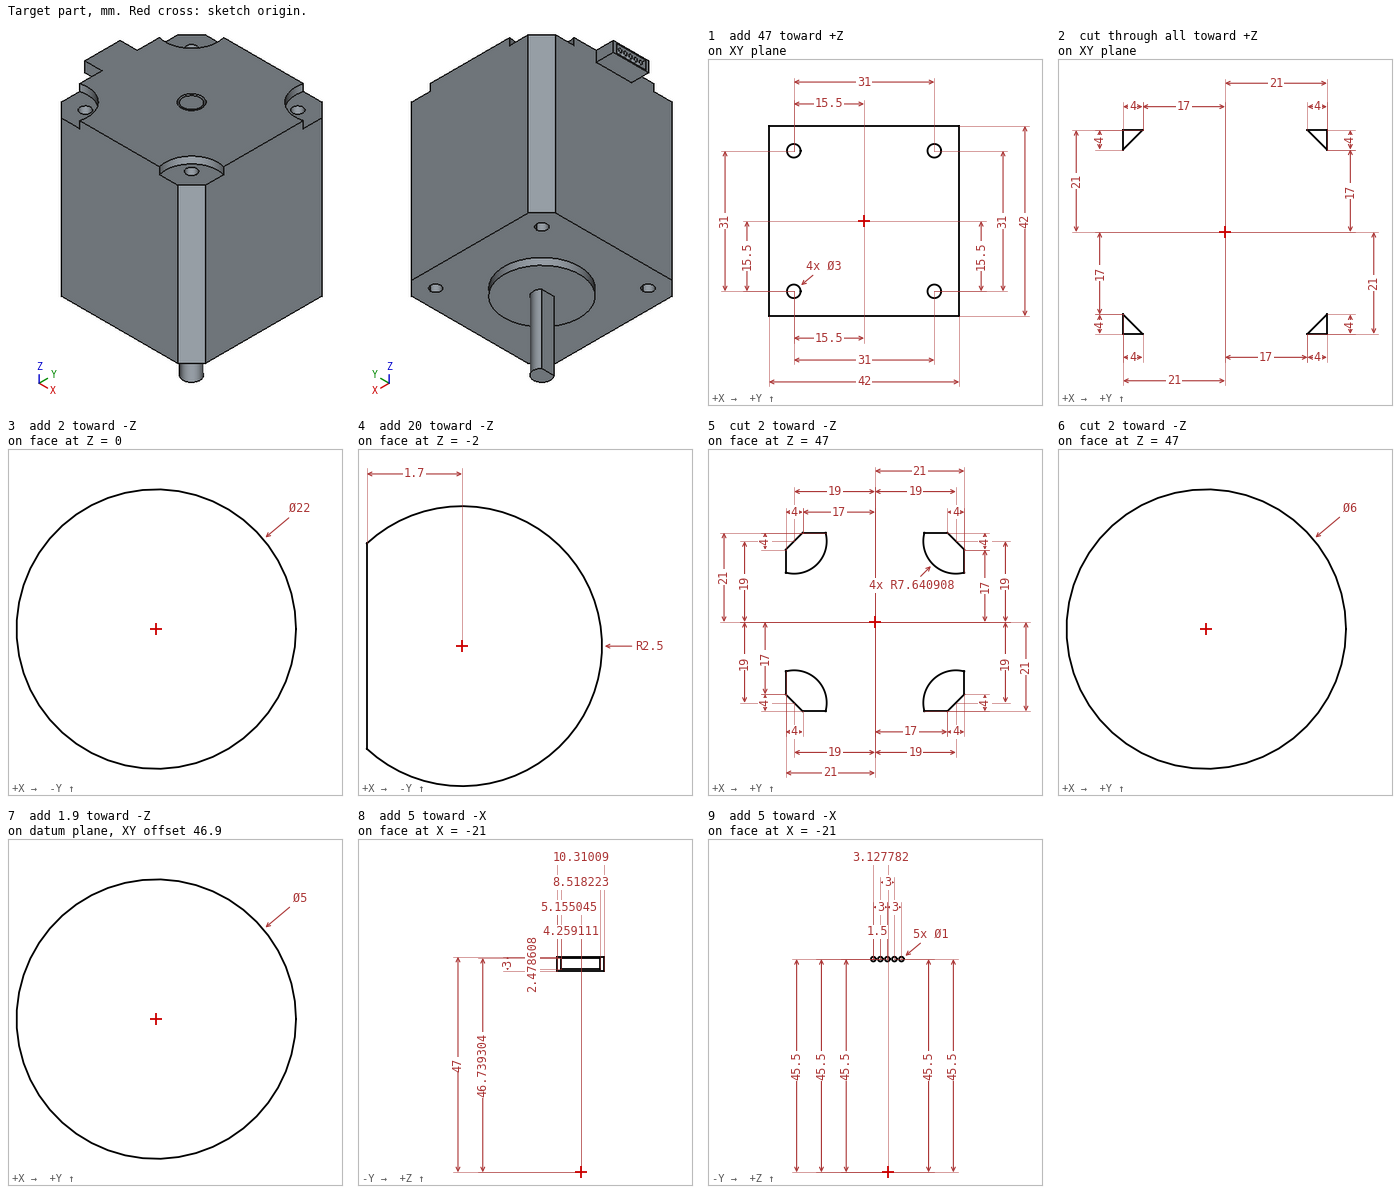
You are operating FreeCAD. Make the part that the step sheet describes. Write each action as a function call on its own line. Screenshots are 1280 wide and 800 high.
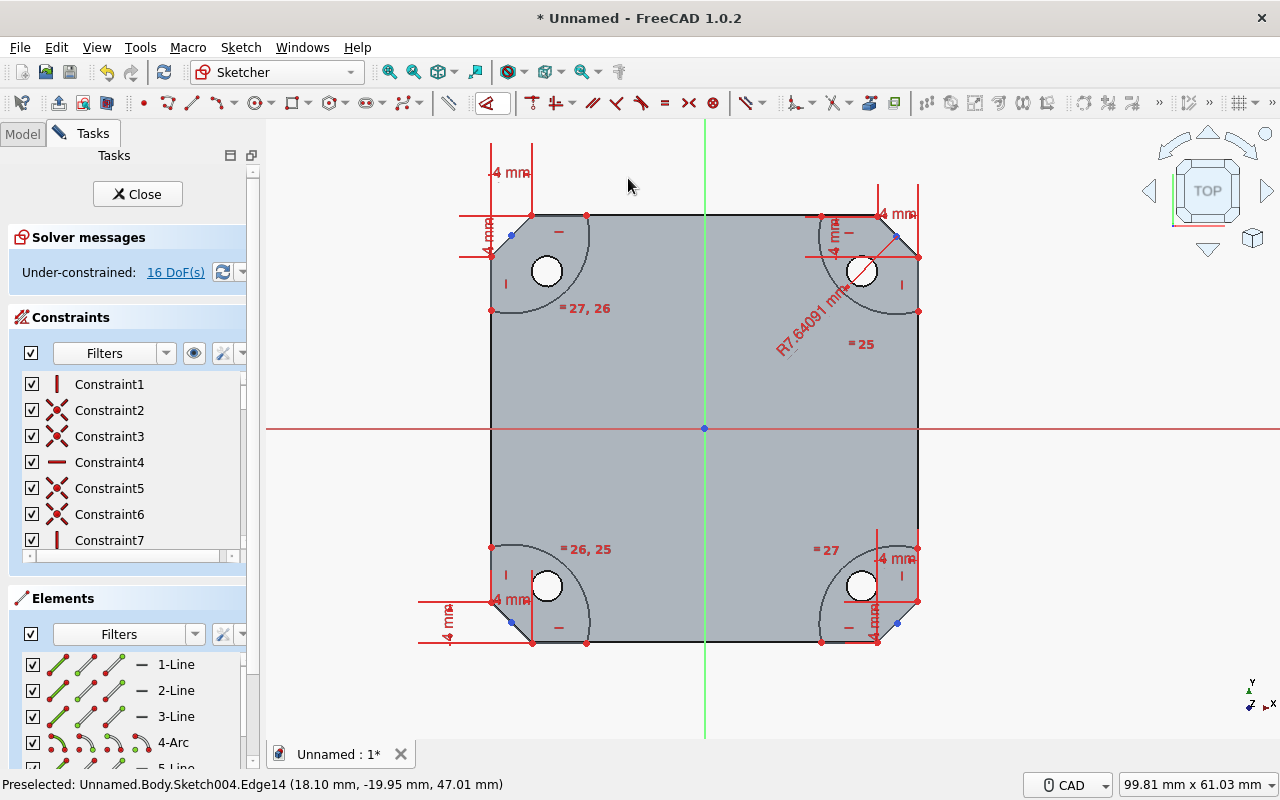
click(918, 311)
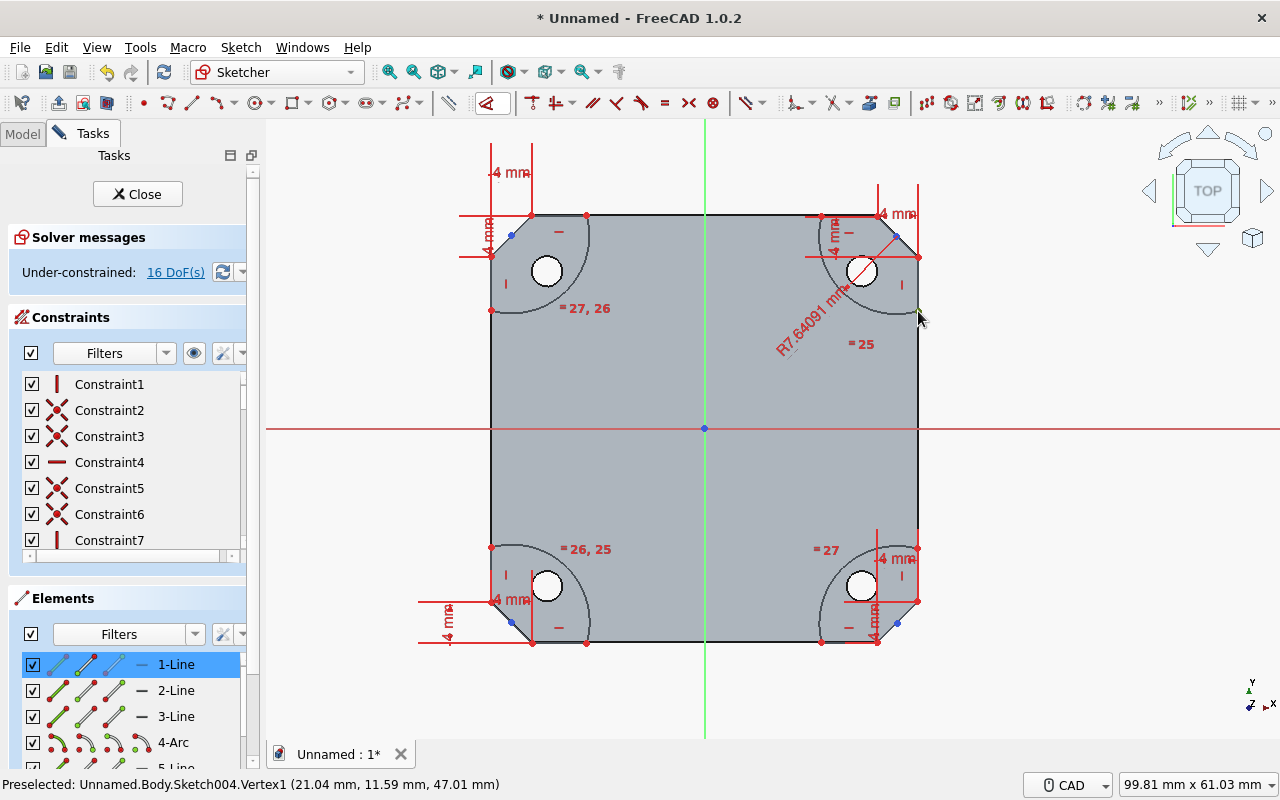
key(l)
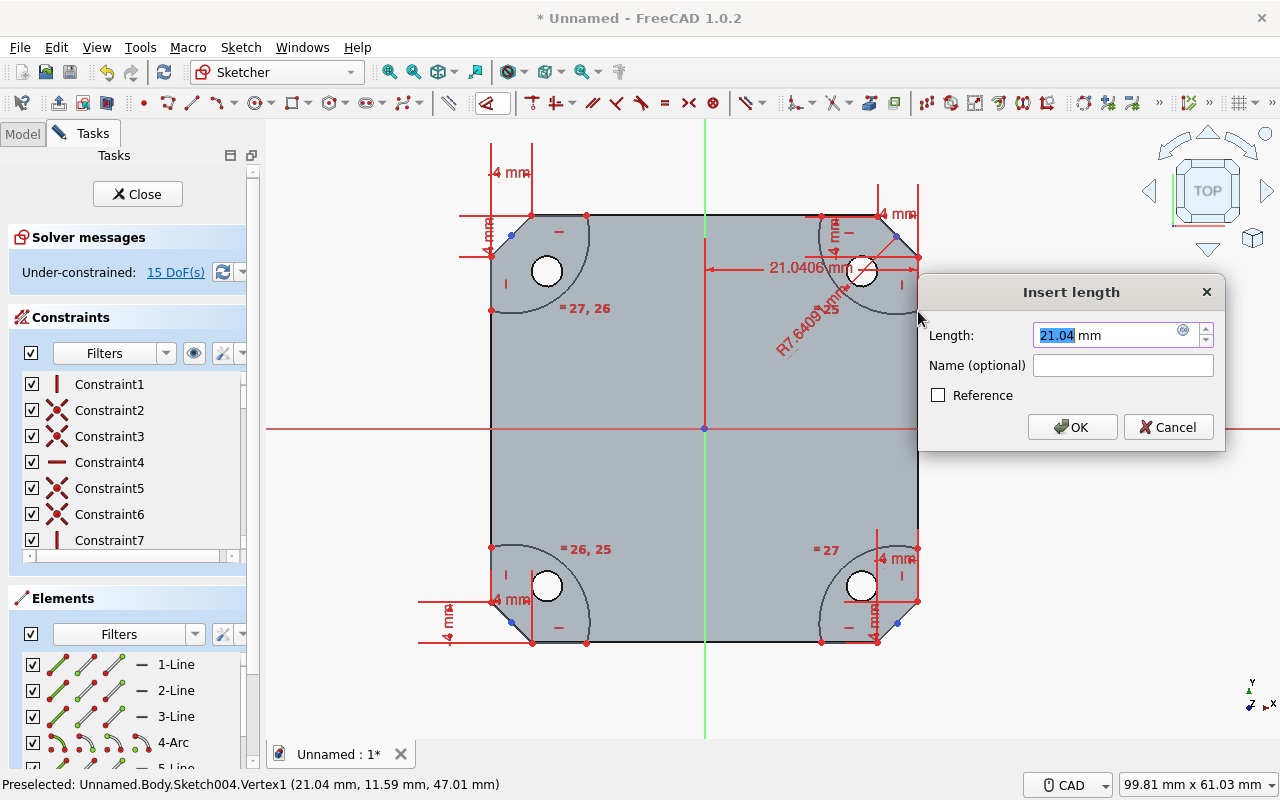
text(21)
key(Return)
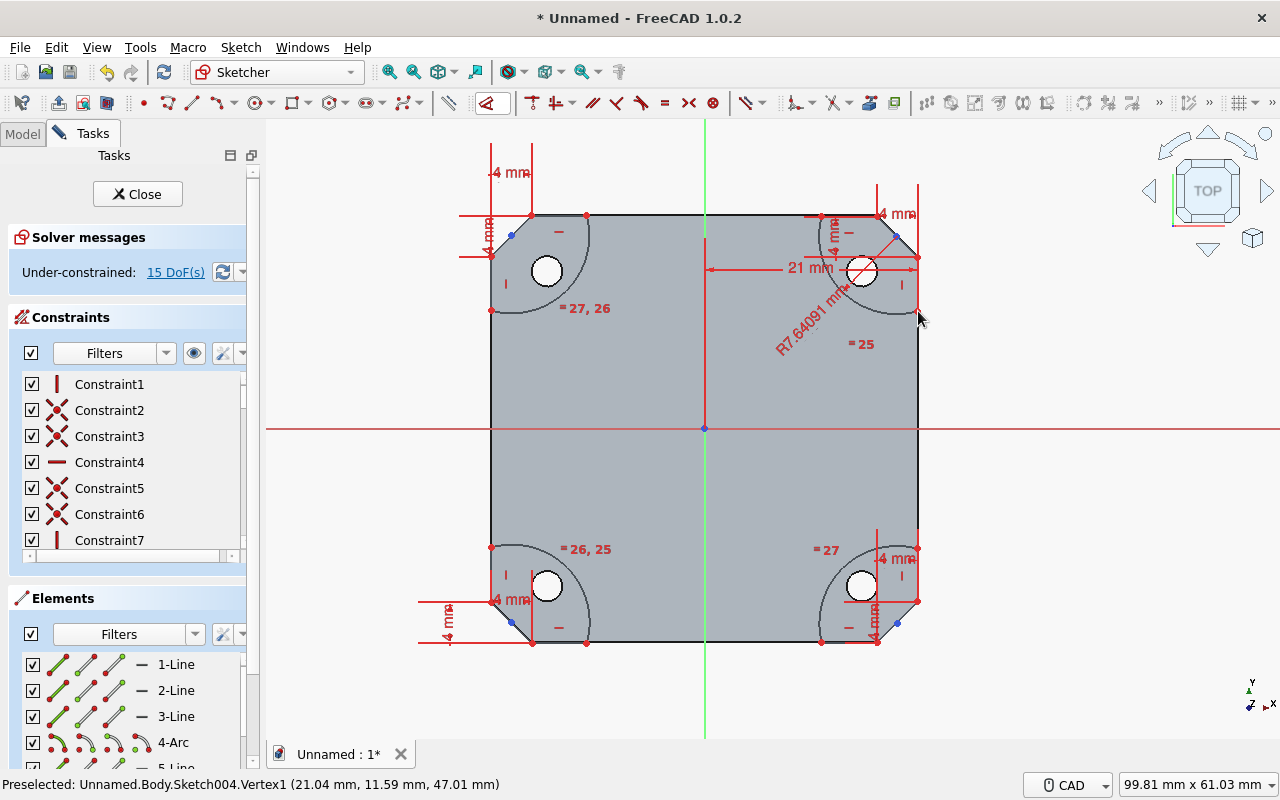
click(918, 257)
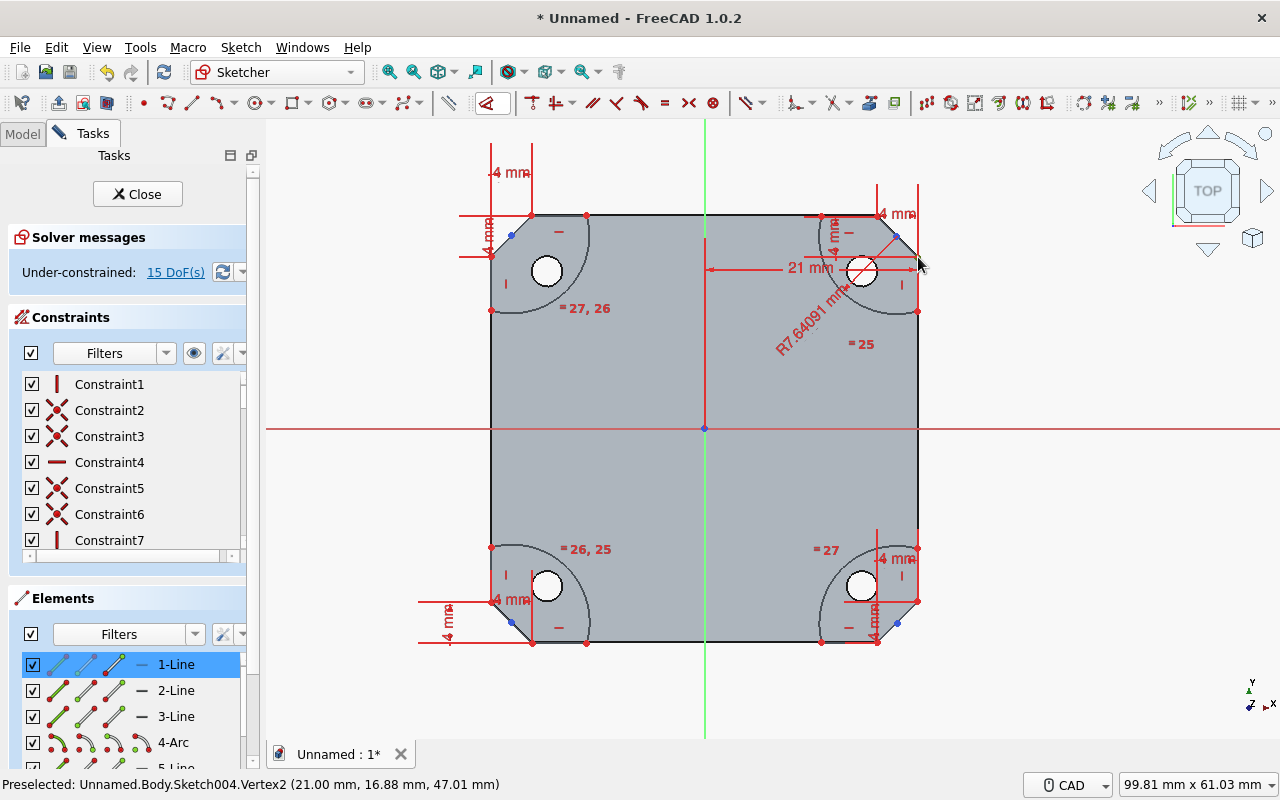
key(i)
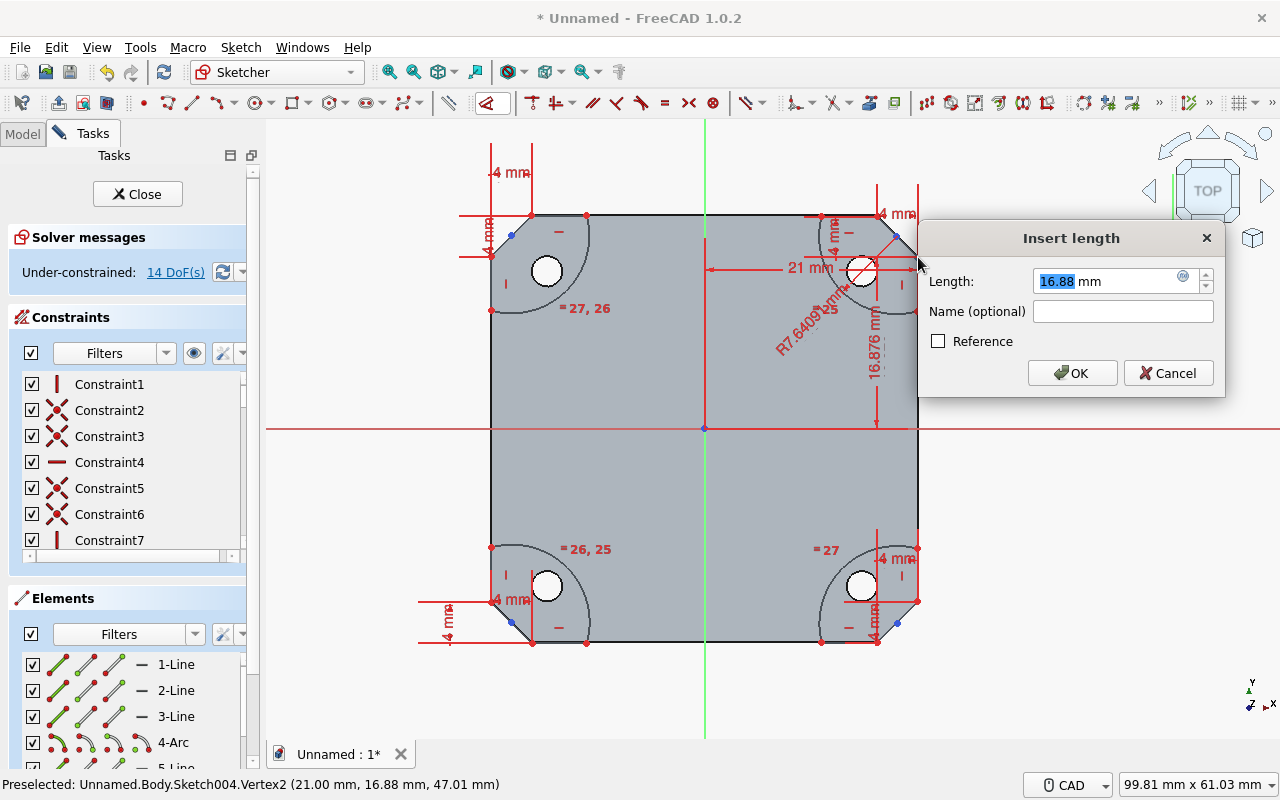
text(17)
key(Return)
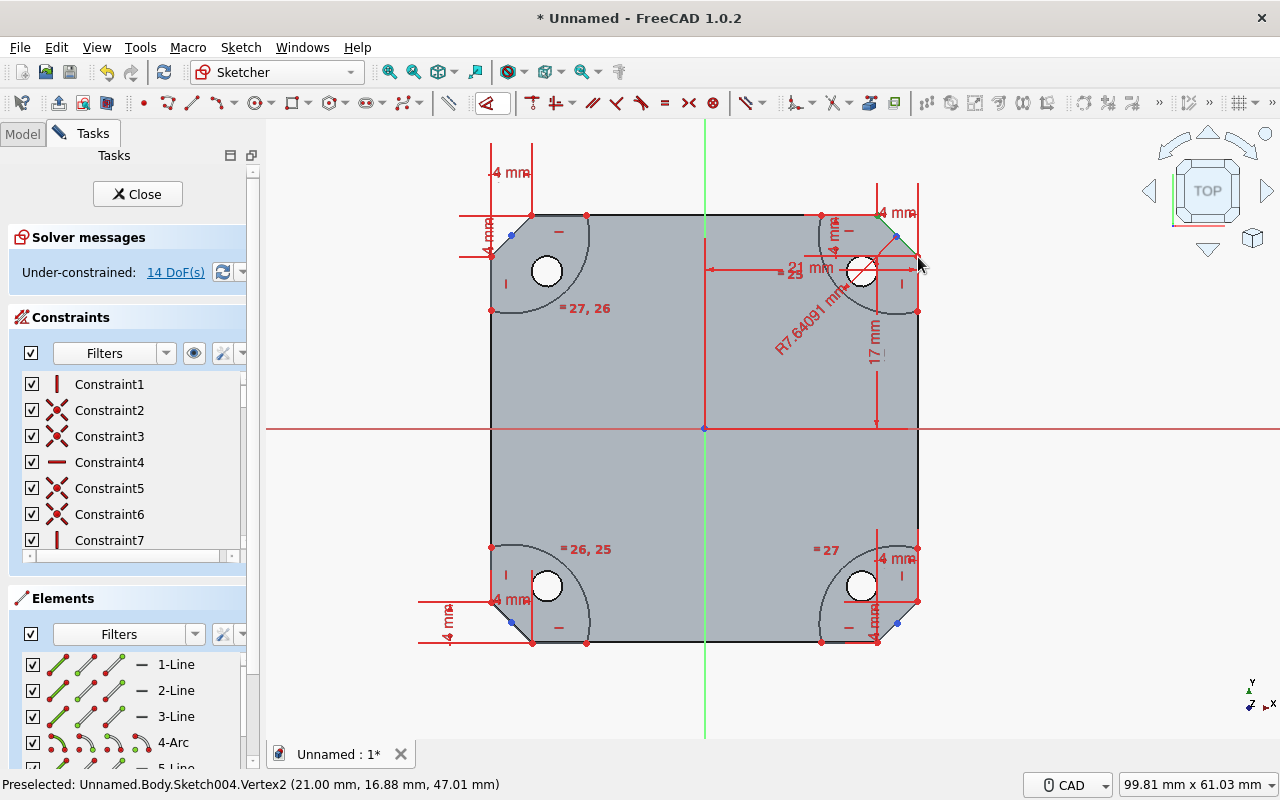
click(491, 547)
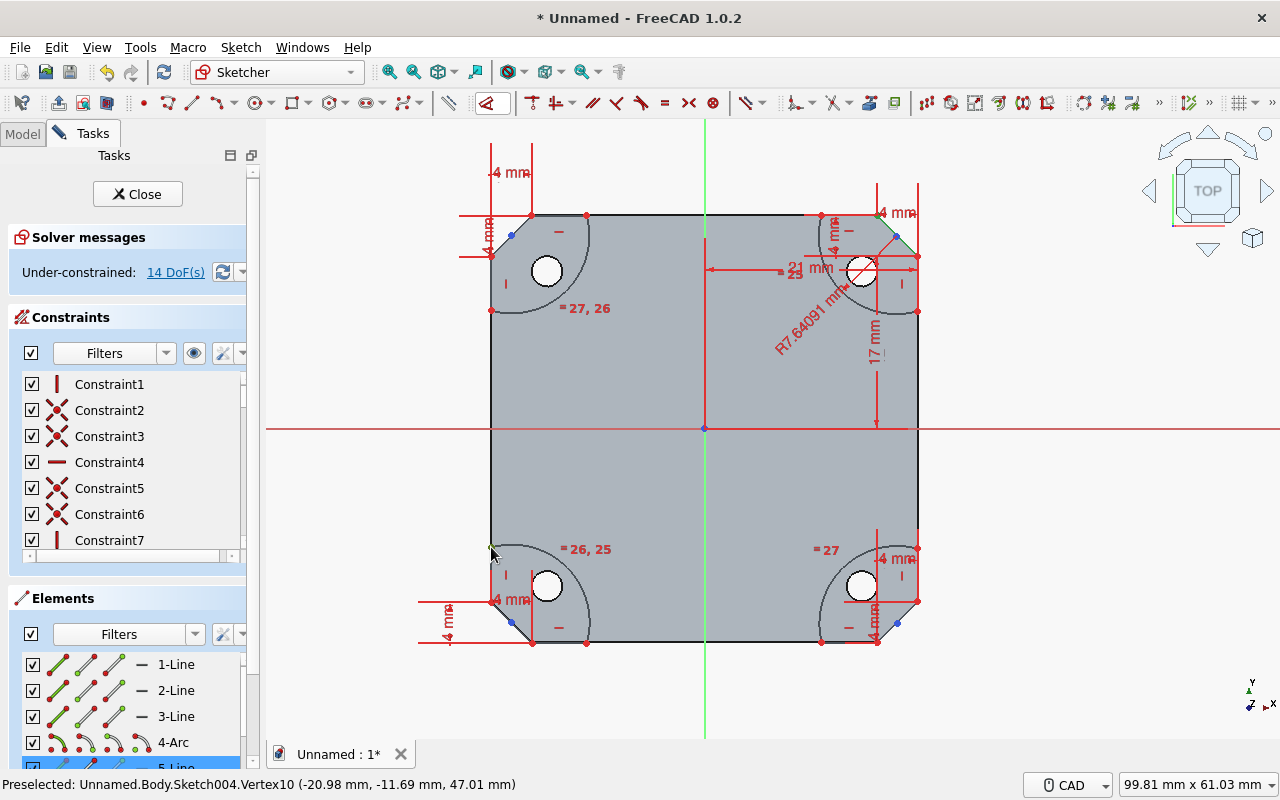
click(504, 104)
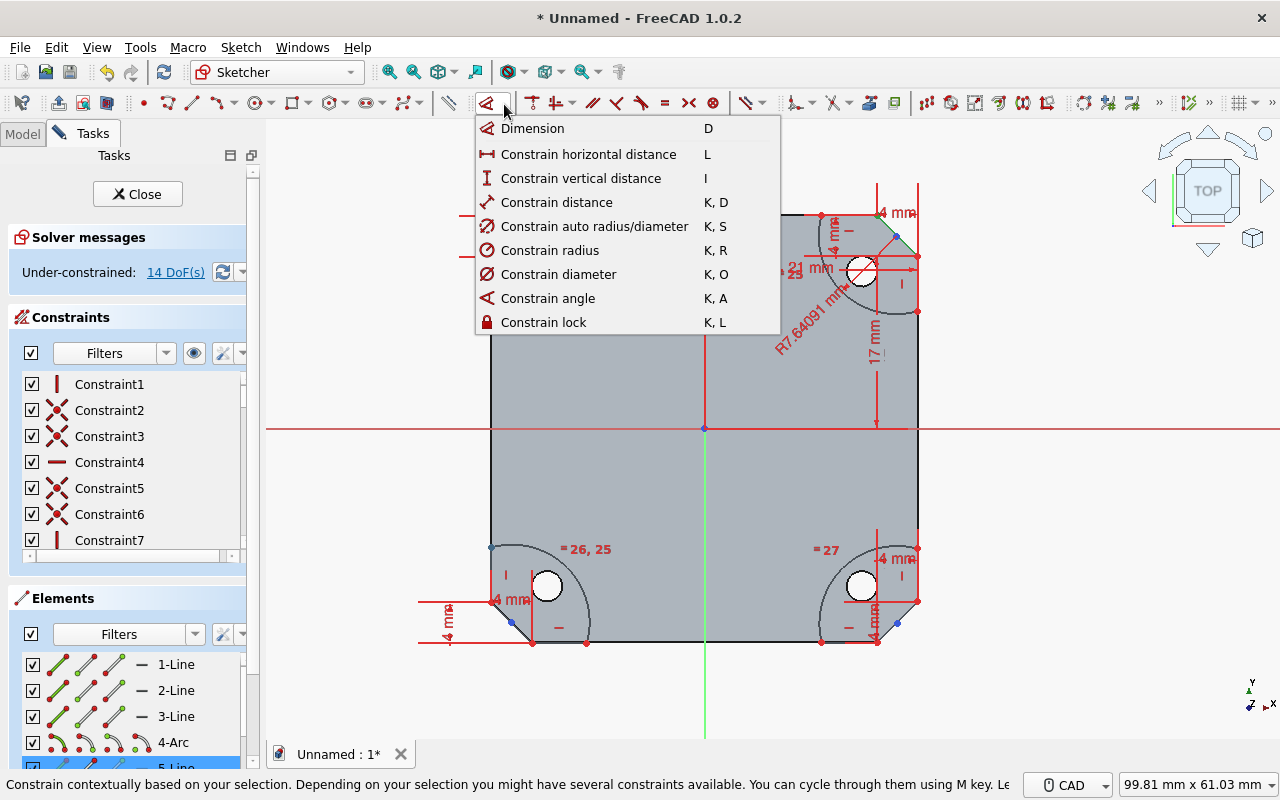
click(628, 154)